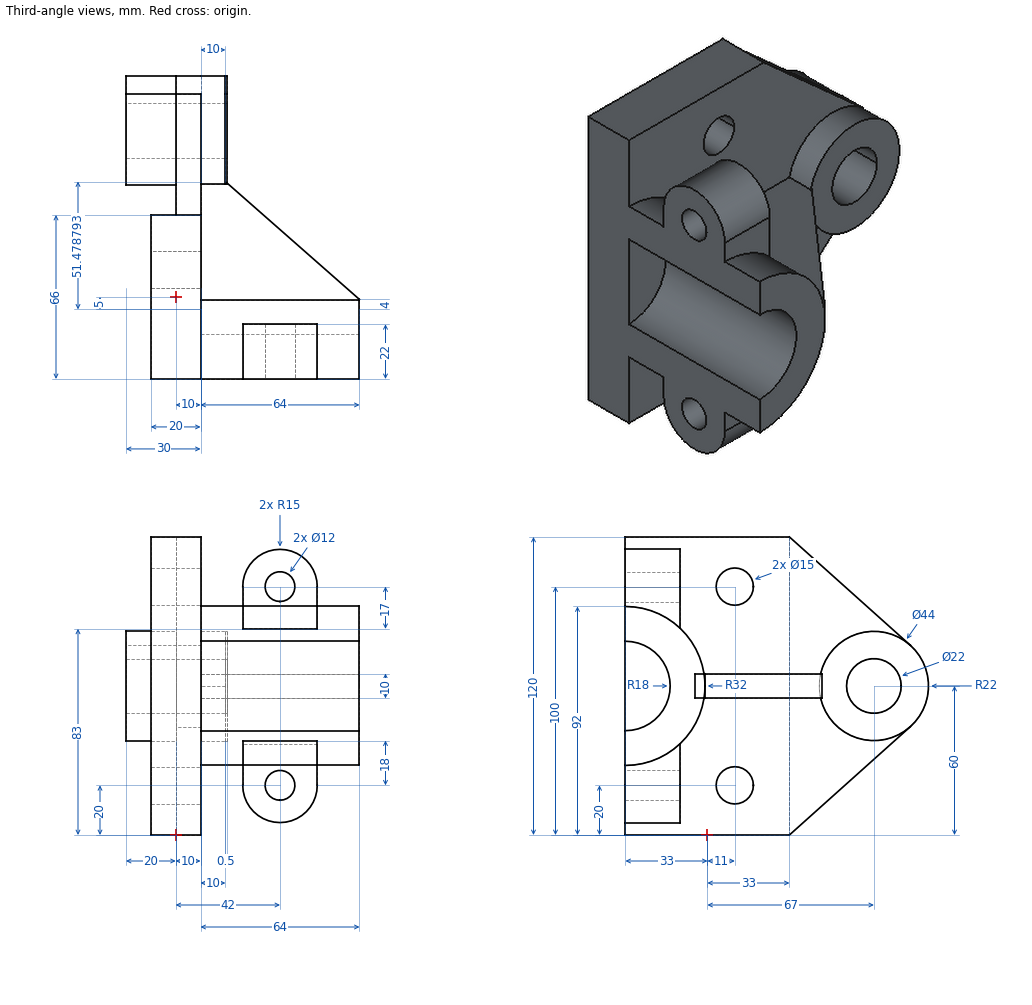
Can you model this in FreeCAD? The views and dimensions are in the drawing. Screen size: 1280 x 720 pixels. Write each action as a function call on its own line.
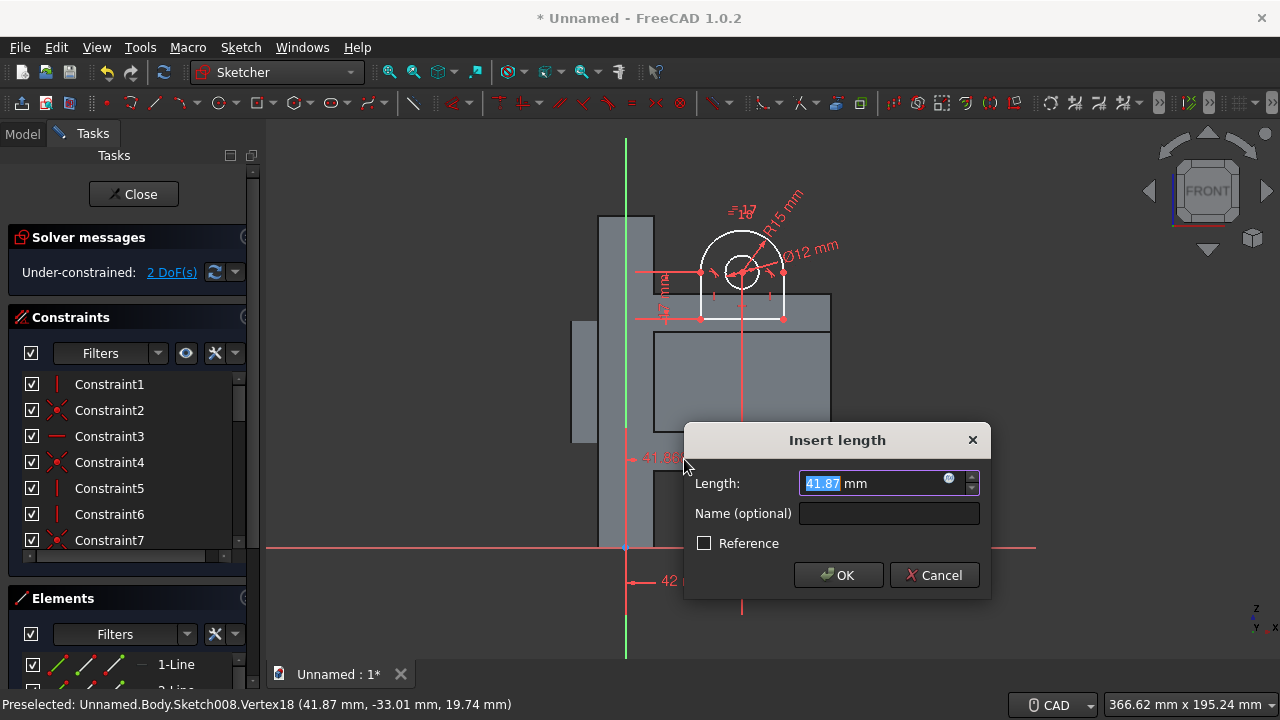
text(42)
key(Return)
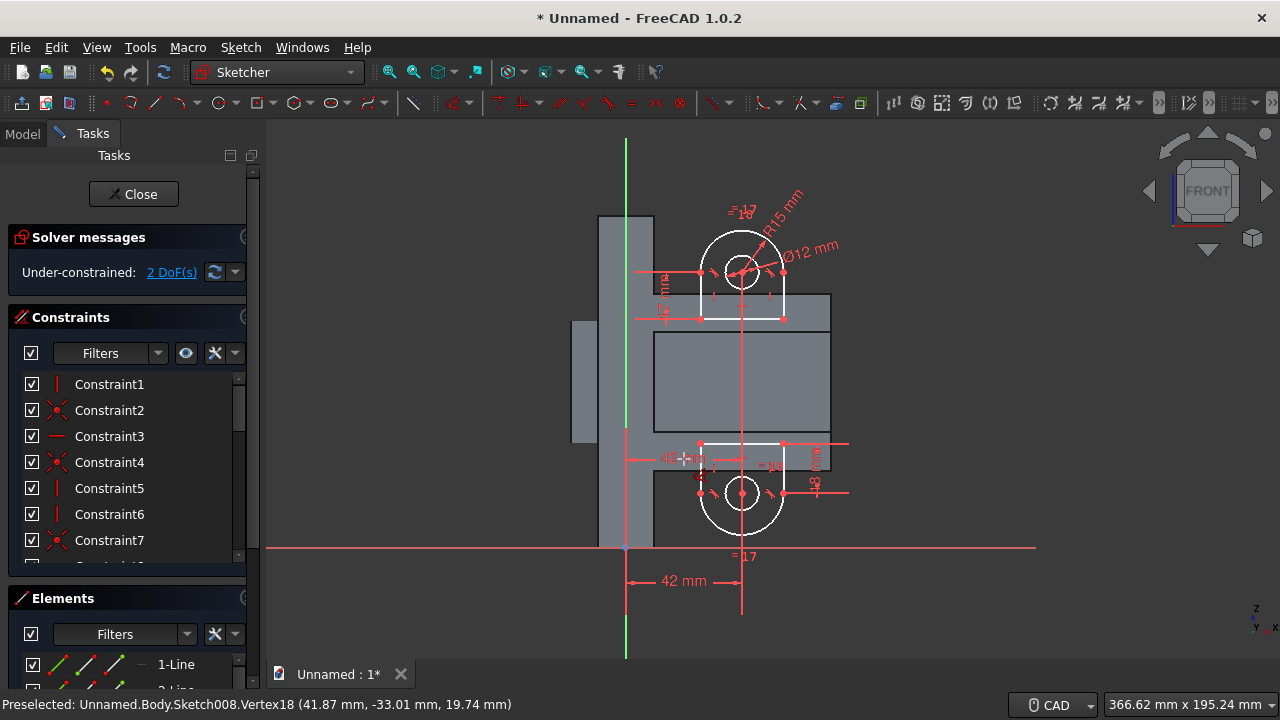
click(742, 493)
click(592, 521)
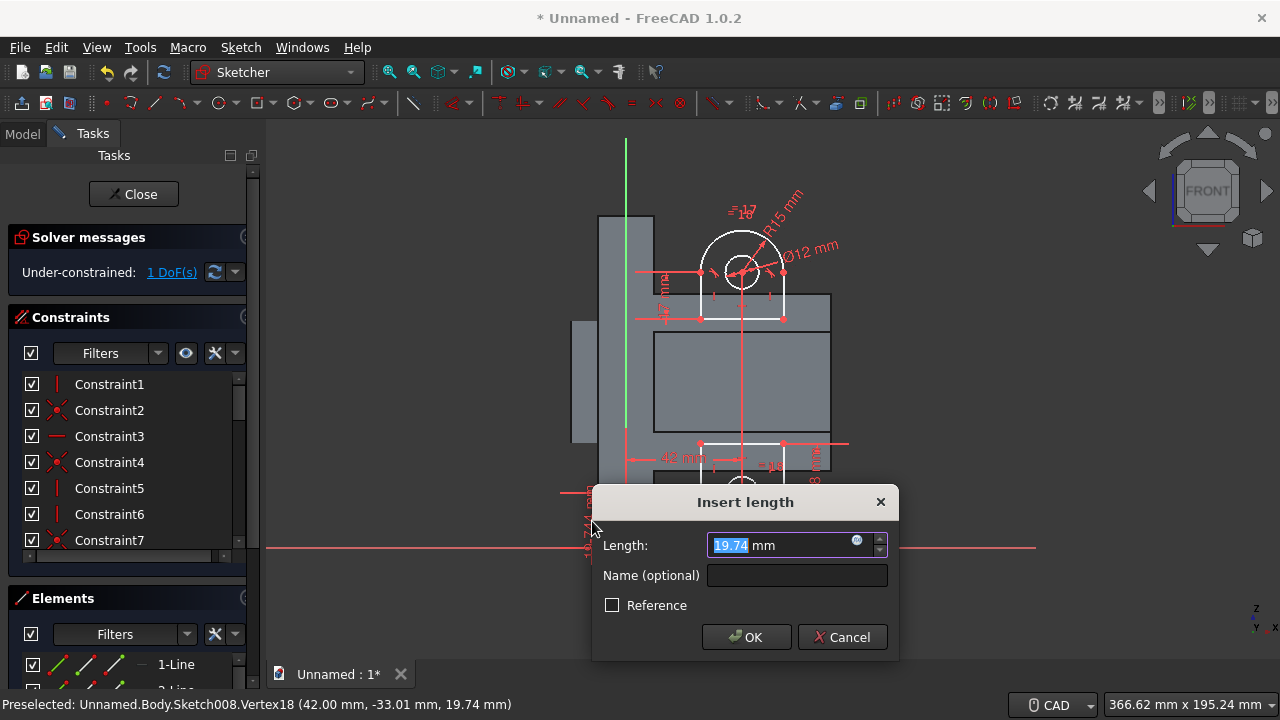
text(20)
key(Return)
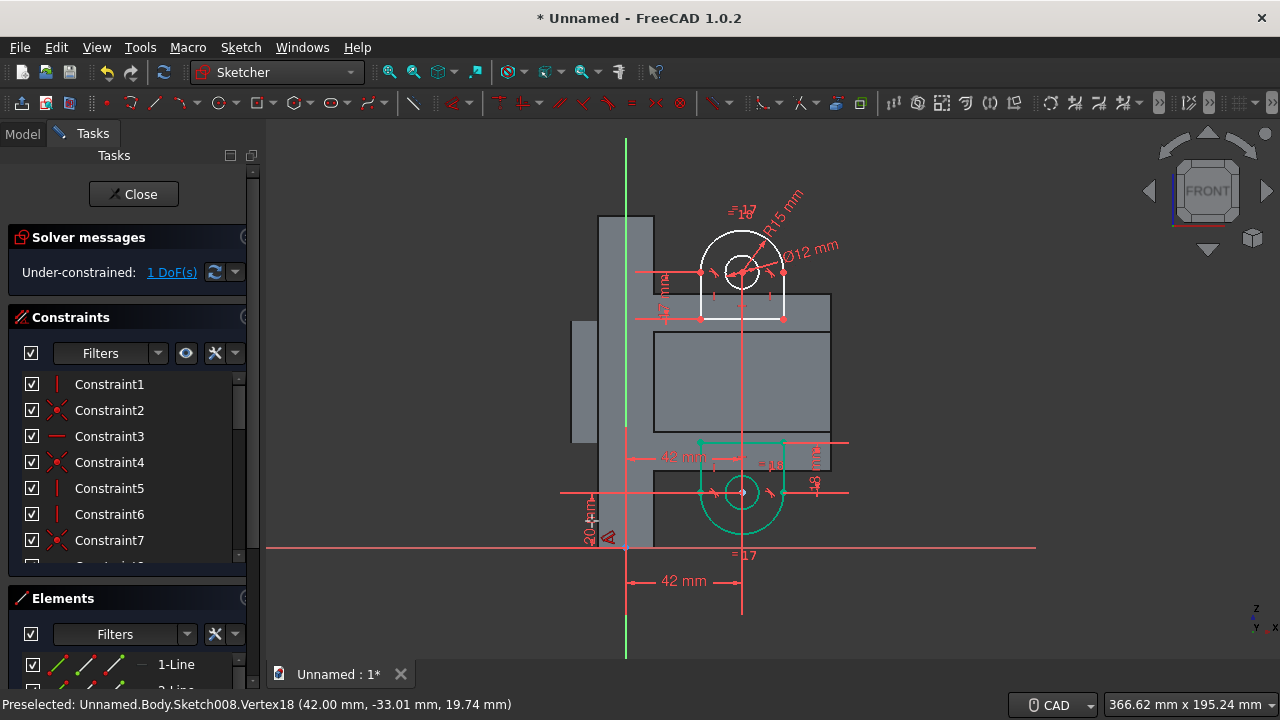
click(701, 319)
click(592, 434)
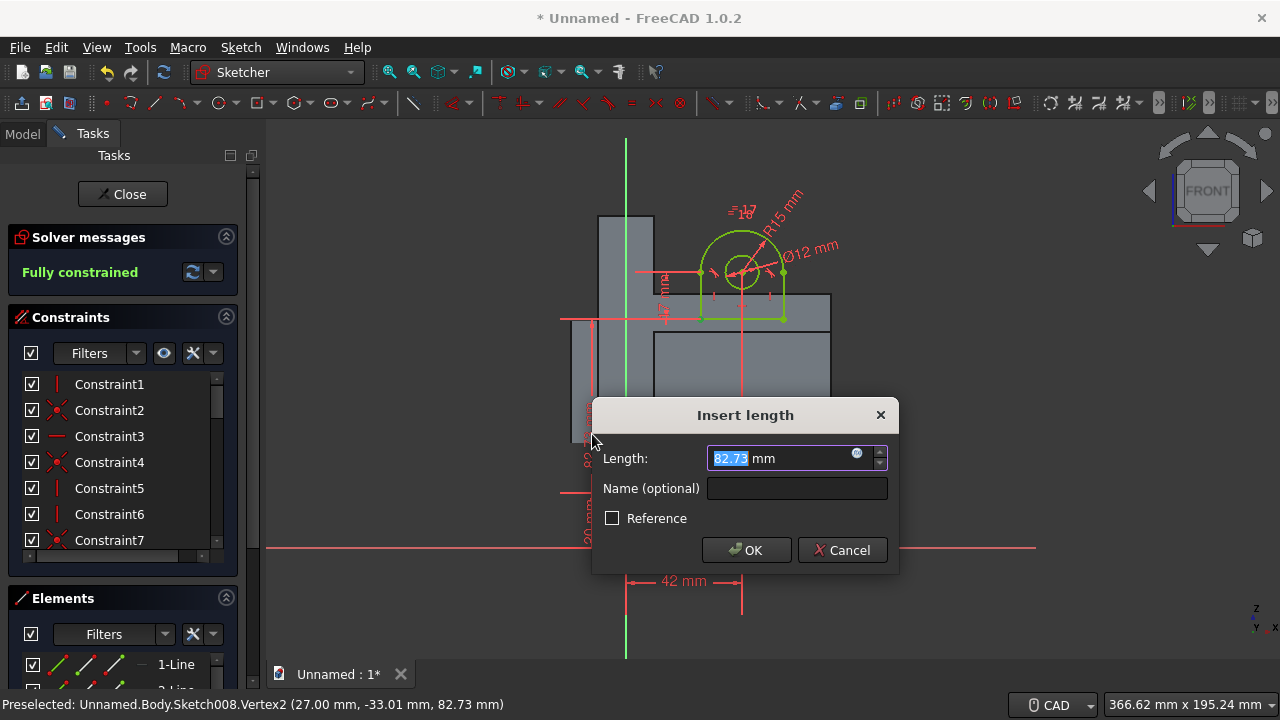
text(83)
key(Return)
key(Escape)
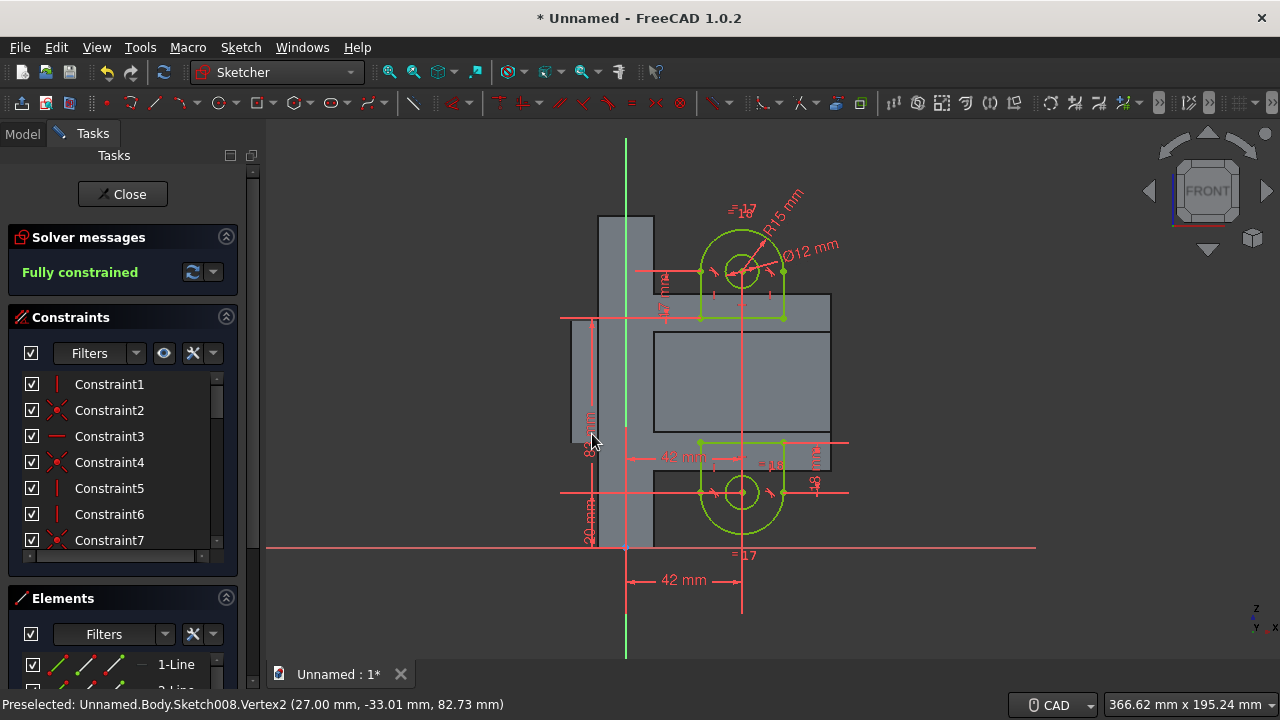
click(123, 194)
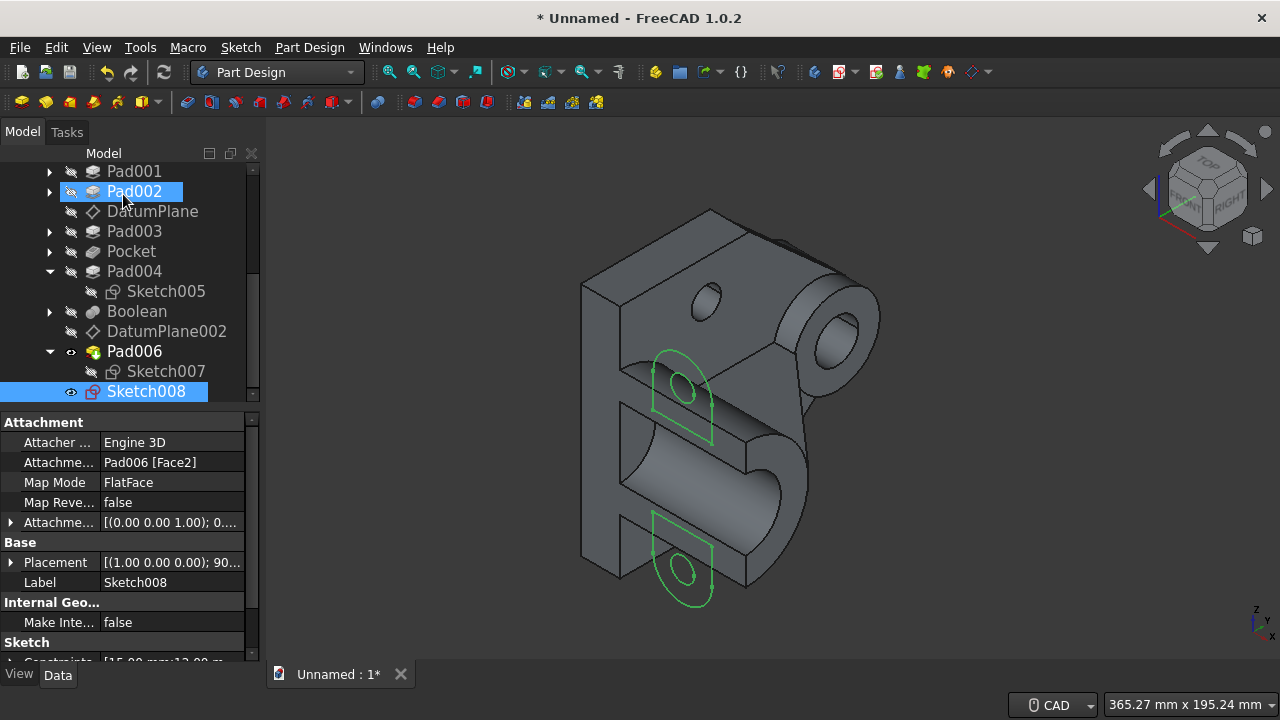
click(22, 102)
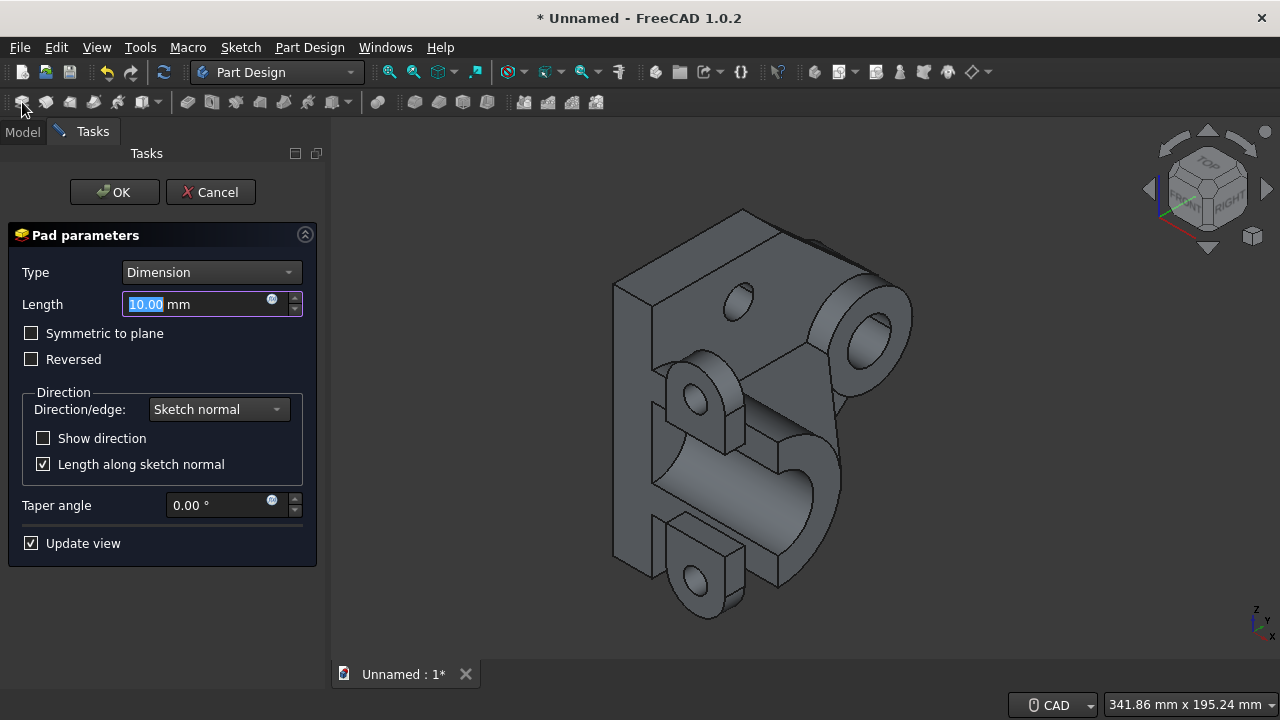
text(22)
key(Tab)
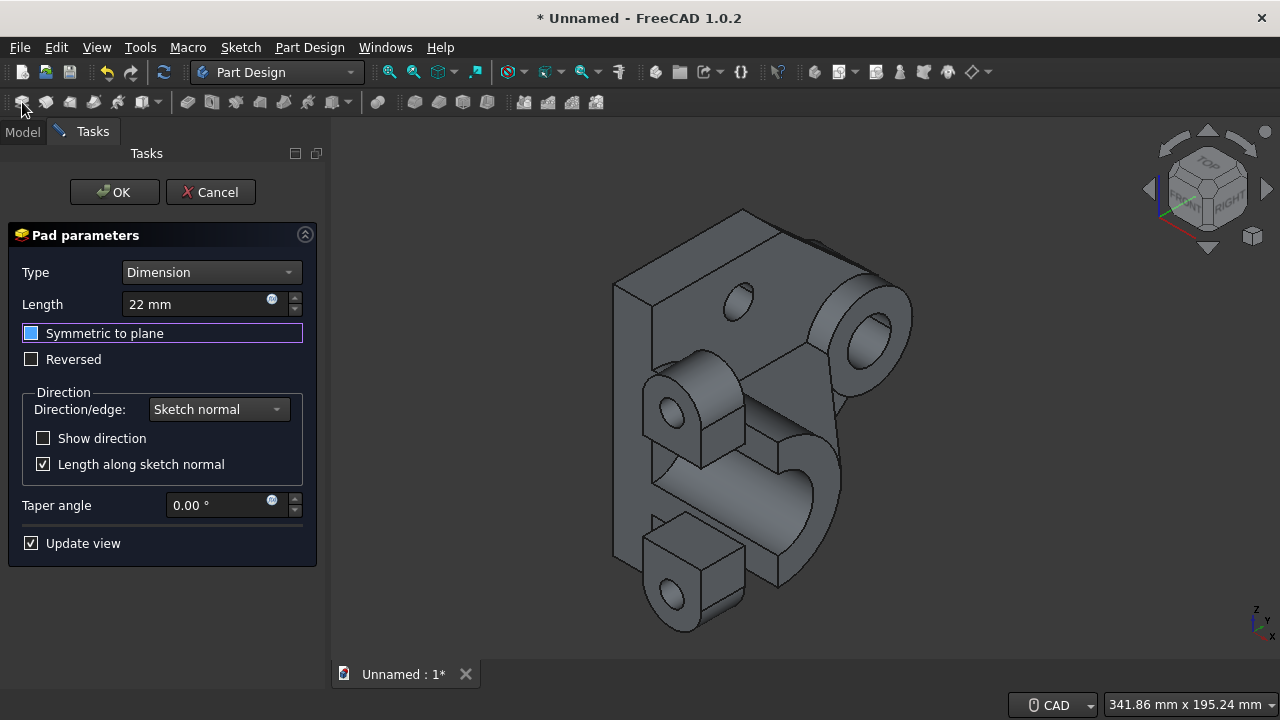
click(30, 359)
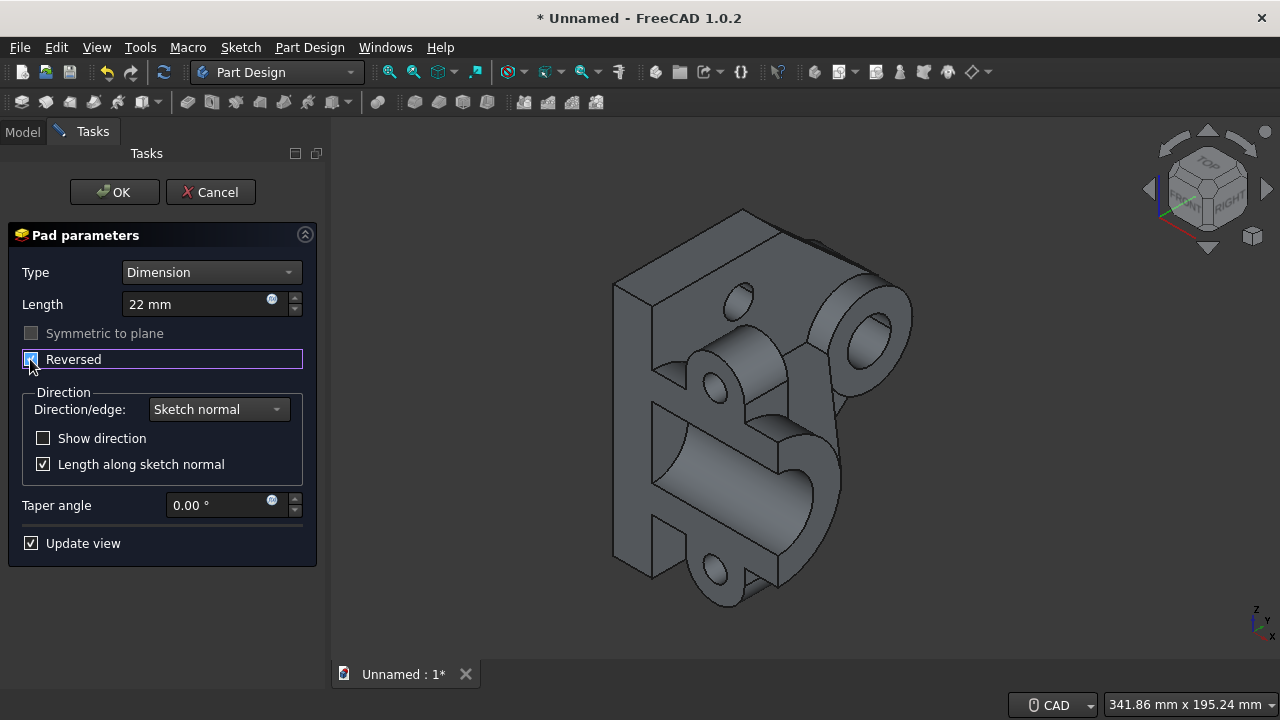
click(115, 192)